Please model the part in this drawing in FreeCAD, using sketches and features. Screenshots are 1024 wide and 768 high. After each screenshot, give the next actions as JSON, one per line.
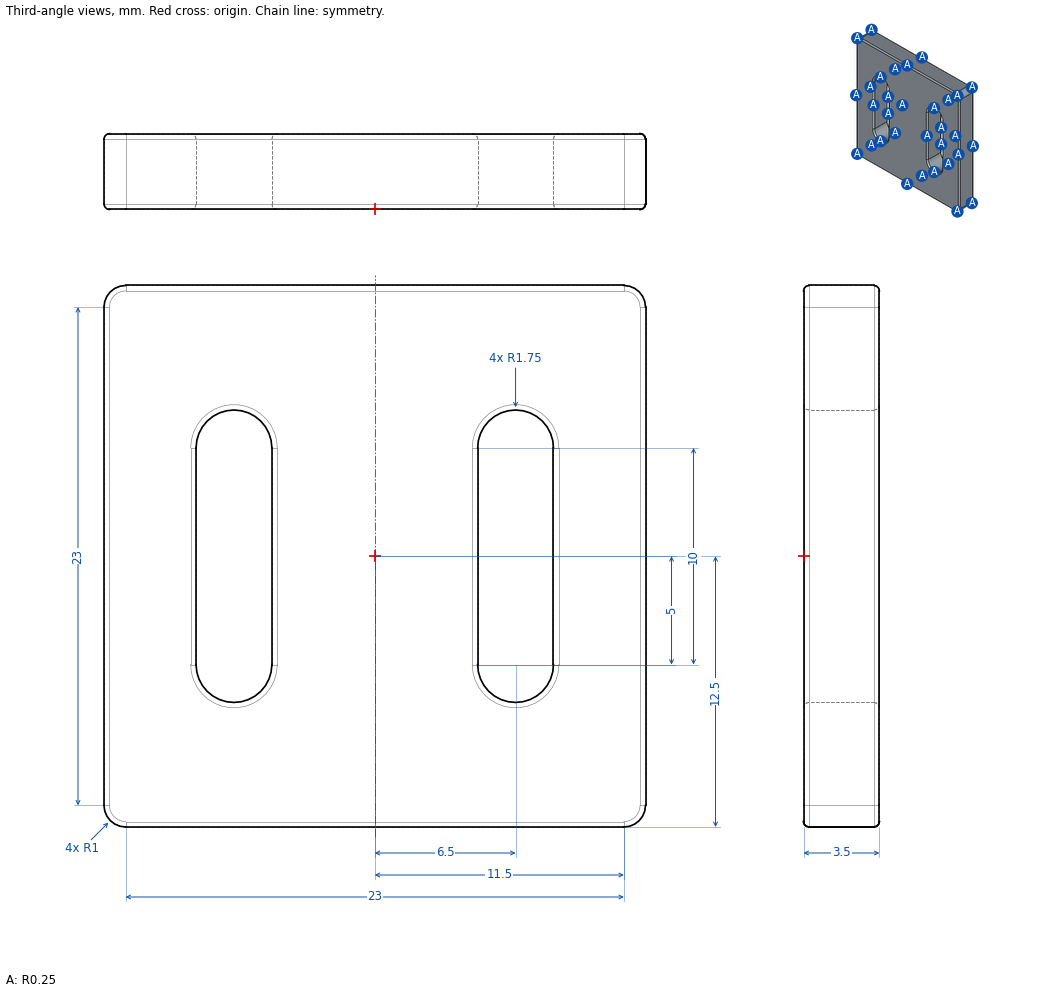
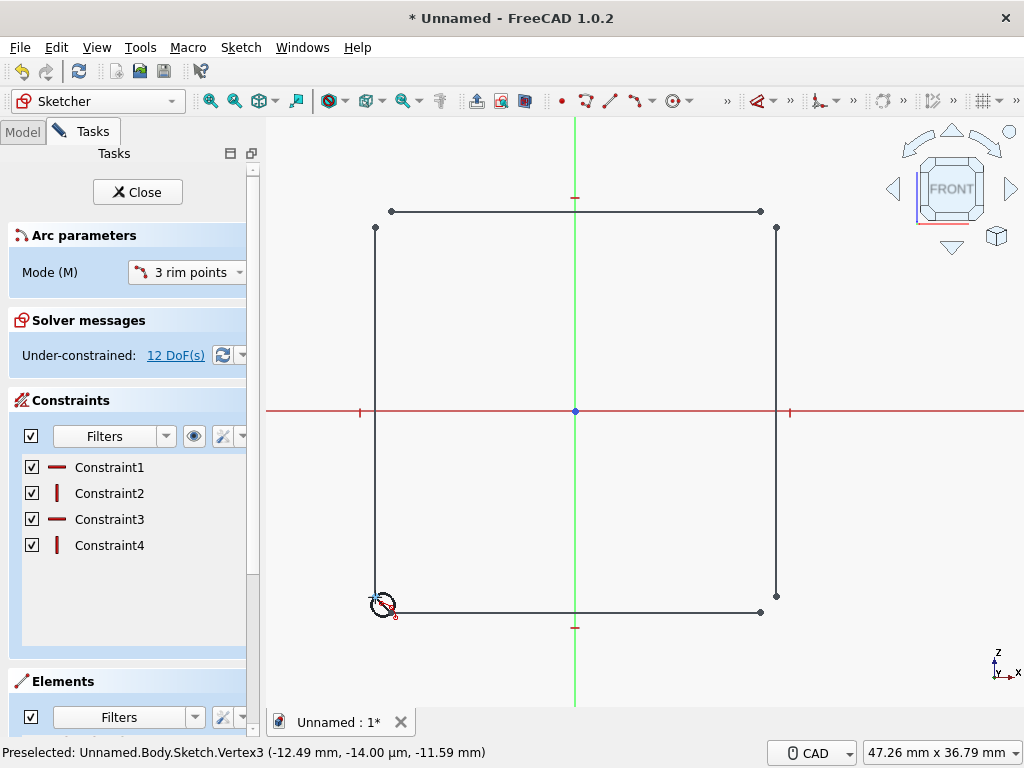
{"action": "scroll", "coordinate": [380, 607], "scroll_direction": "up", "scroll_amount": 7}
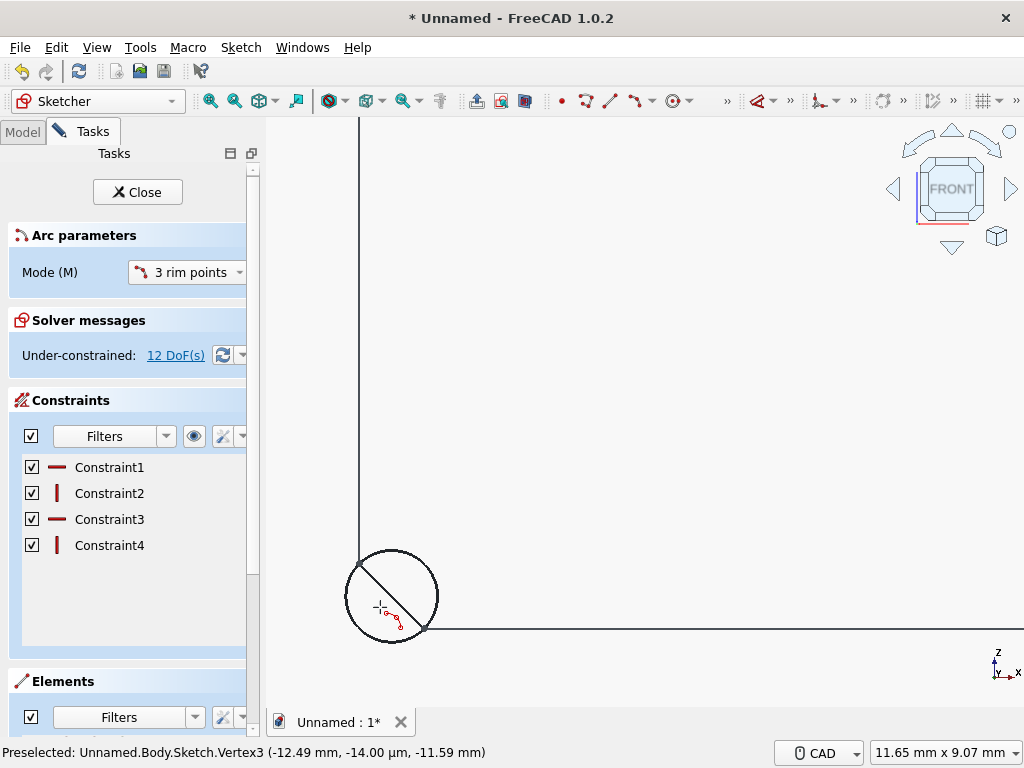
{"action": "left_click", "coordinate": [378, 604]}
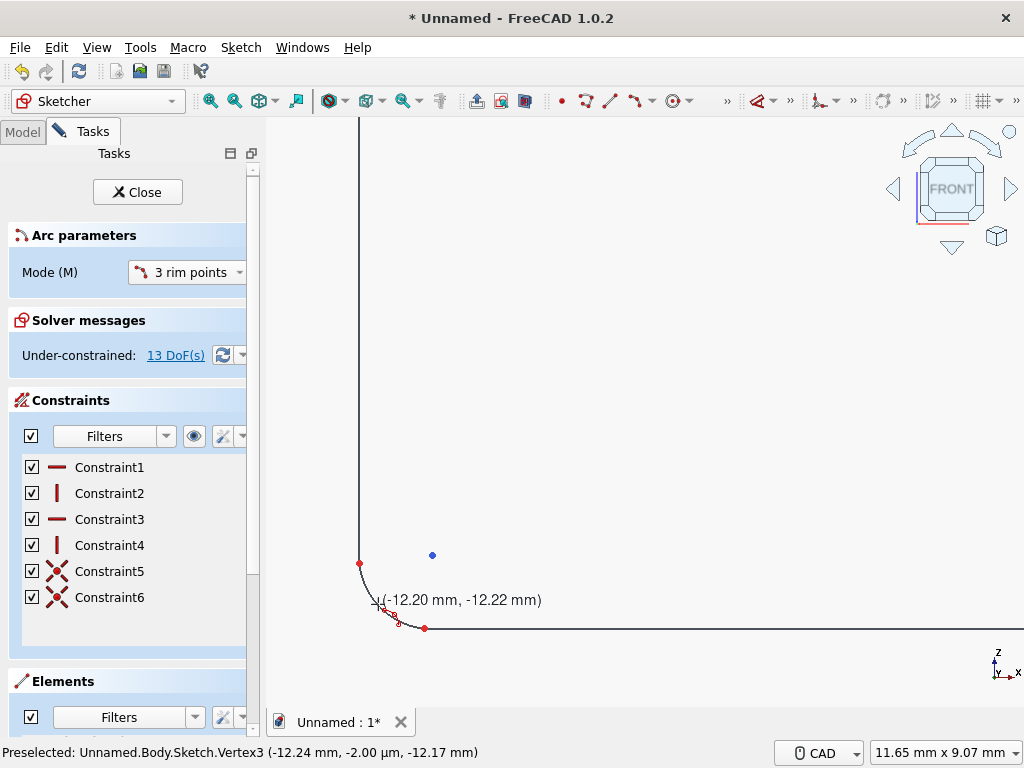
{"action": "scroll", "coordinate": [382, 609], "scroll_direction": "down", "scroll_amount": 7}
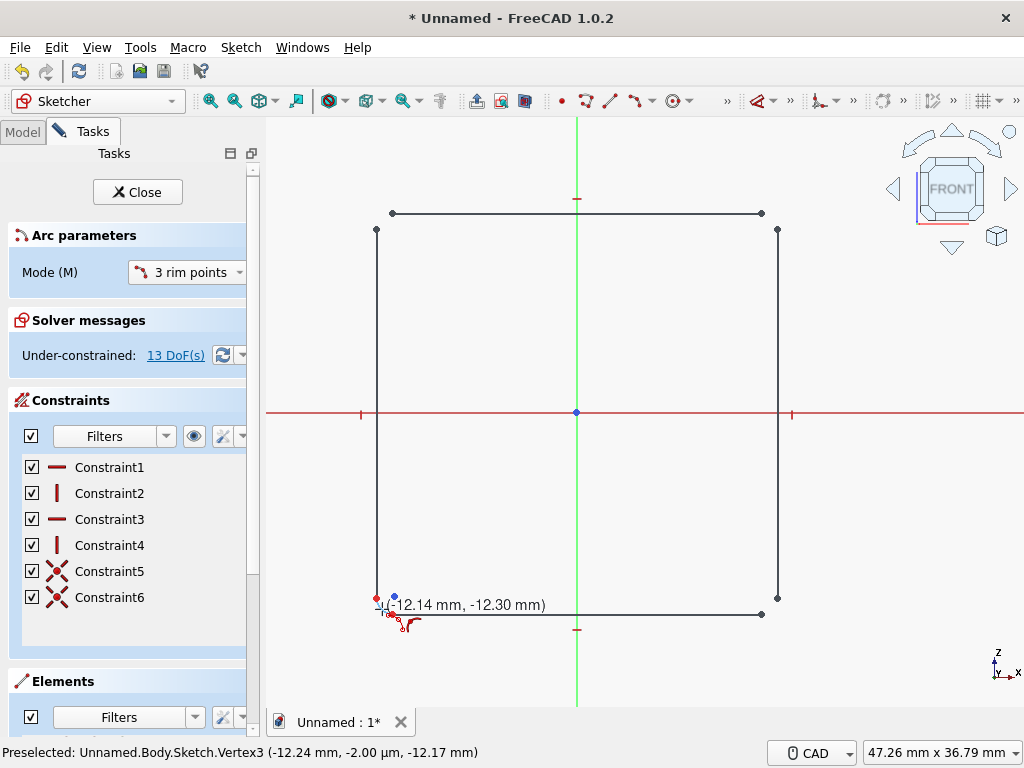
{"action": "left_click", "coordinate": [377, 230]}
{"action": "left_click", "coordinate": [393, 214]}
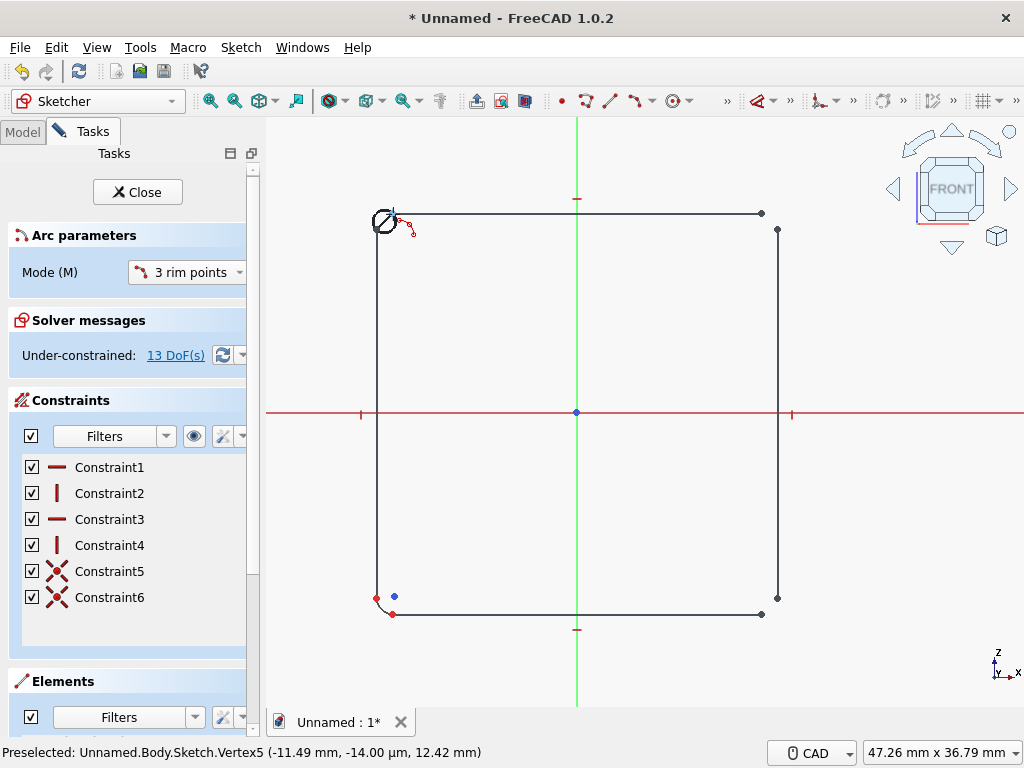
{"action": "scroll", "coordinate": [381, 217], "scroll_direction": "up", "scroll_amount": 7}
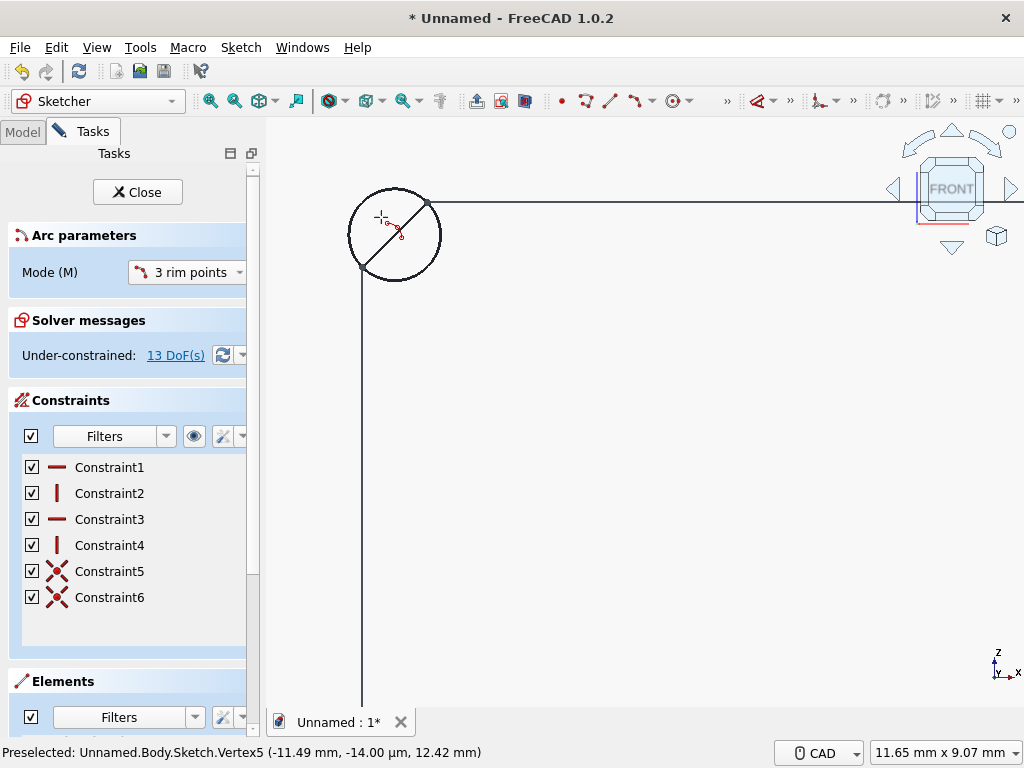
{"action": "left_click", "coordinate": [381, 216]}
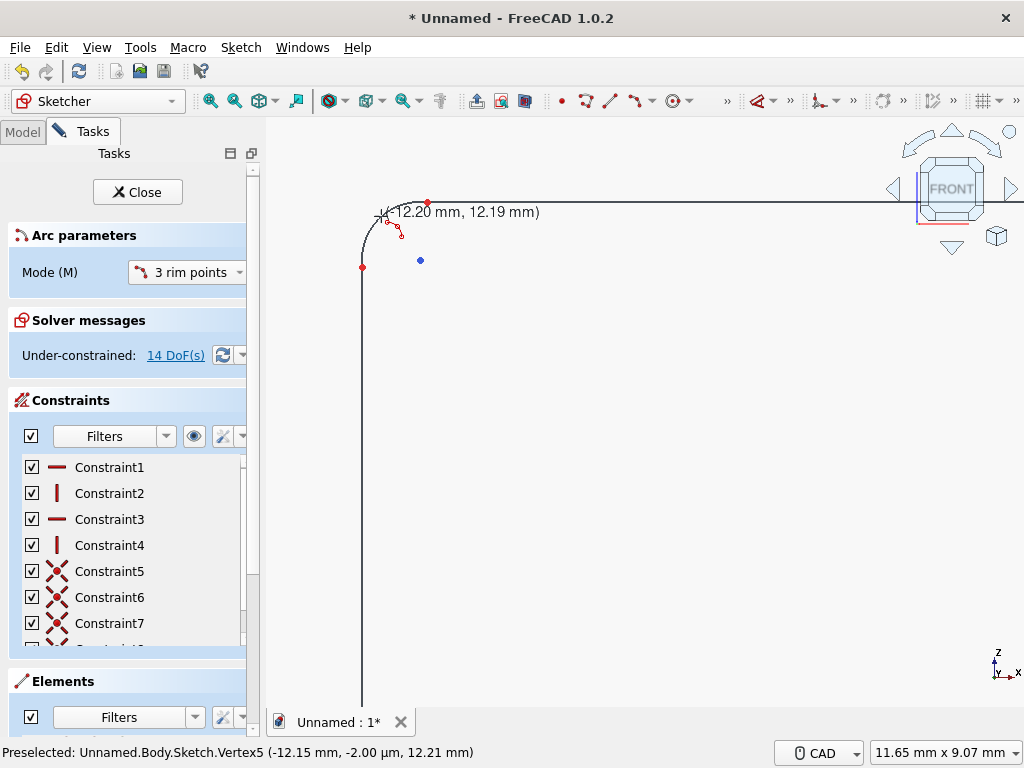
{"action": "scroll", "coordinate": [381, 216], "scroll_direction": "down", "scroll_amount": 7}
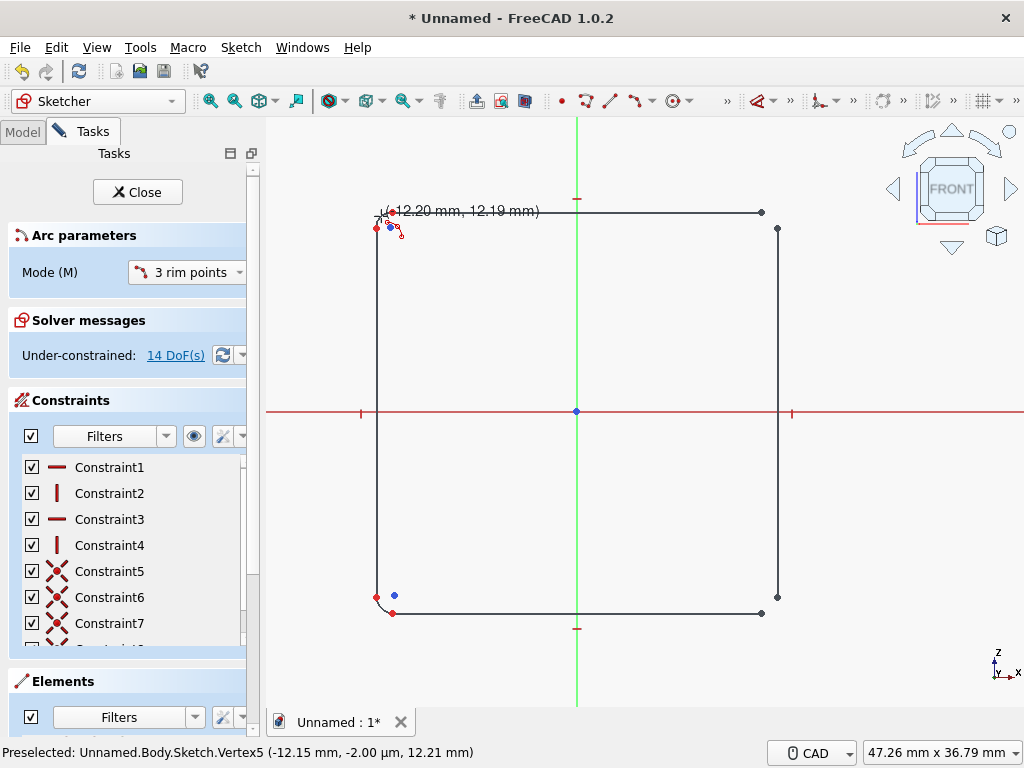
{"action": "left_click", "coordinate": [762, 213]}
{"action": "left_click", "coordinate": [778, 229]}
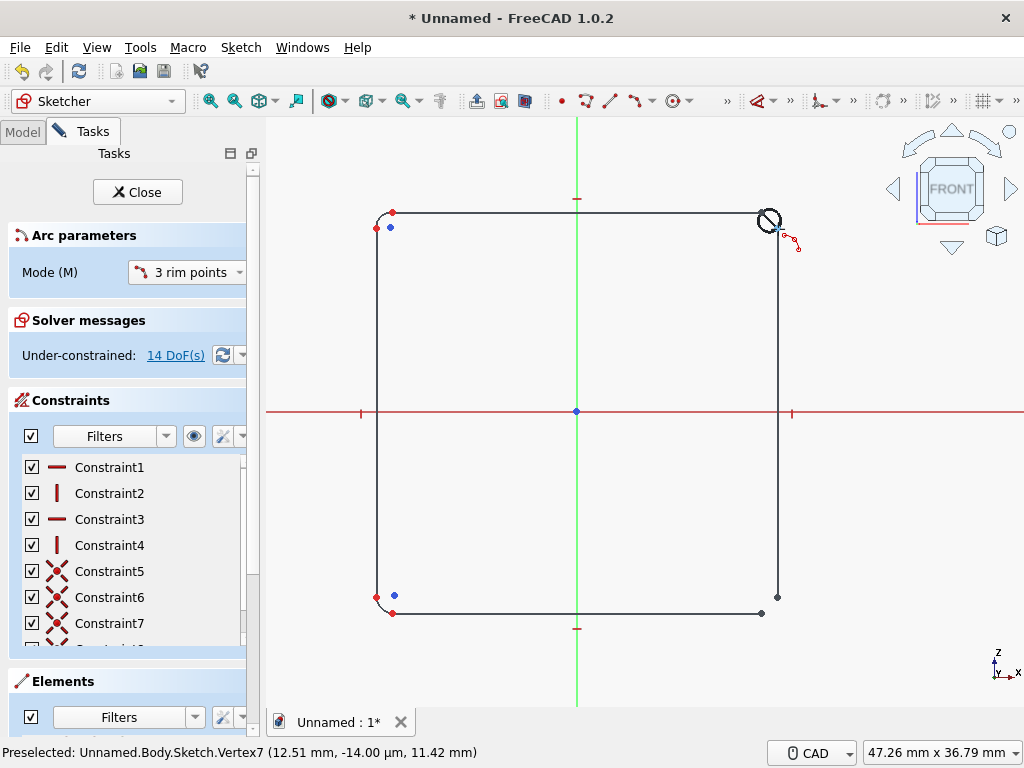
{"action": "scroll", "coordinate": [773, 216], "scroll_direction": "up", "scroll_amount": 7}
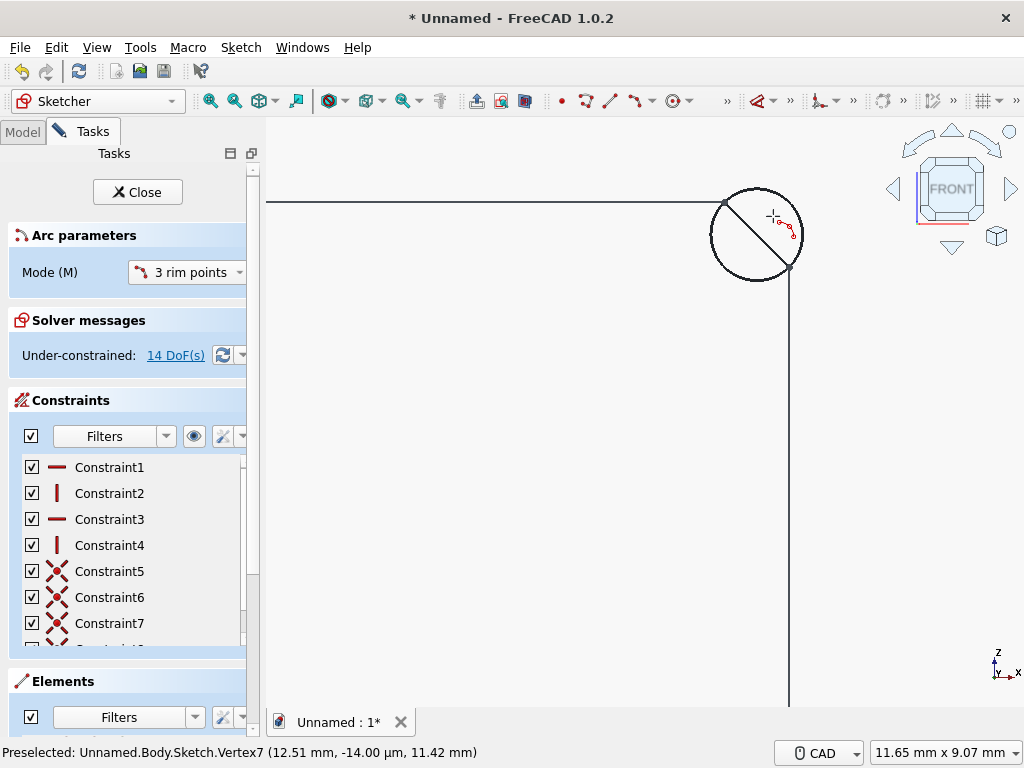
{"action": "left_click", "coordinate": [769, 216]}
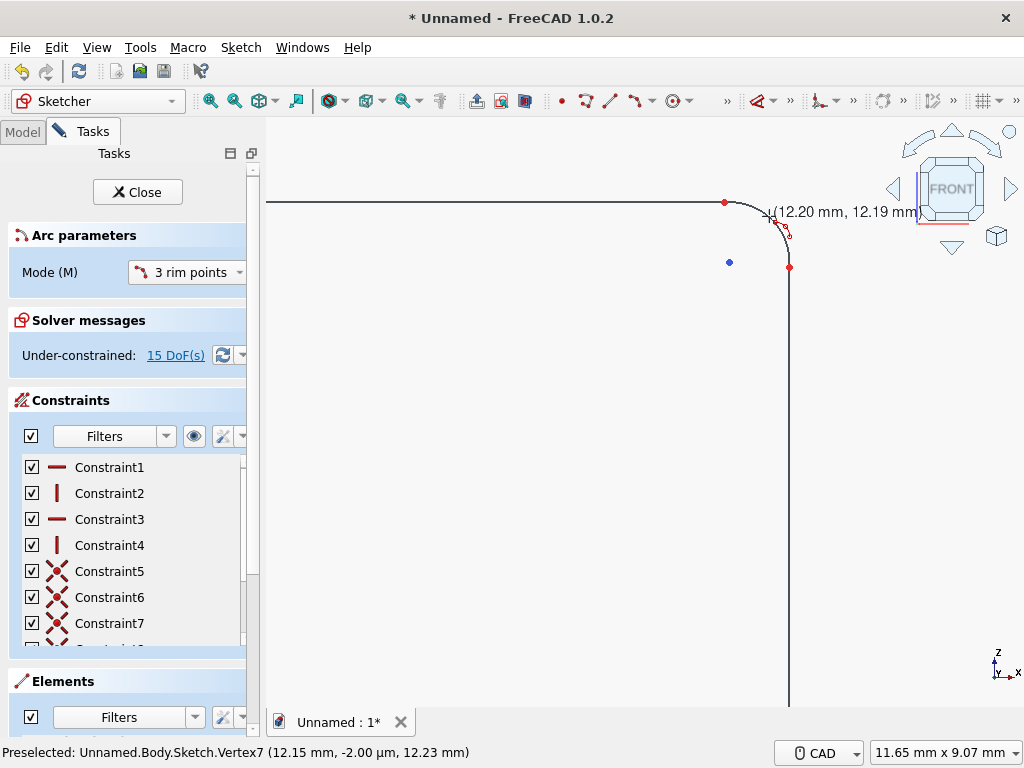
{"action": "scroll", "coordinate": [773, 216], "scroll_direction": "down", "scroll_amount": 7}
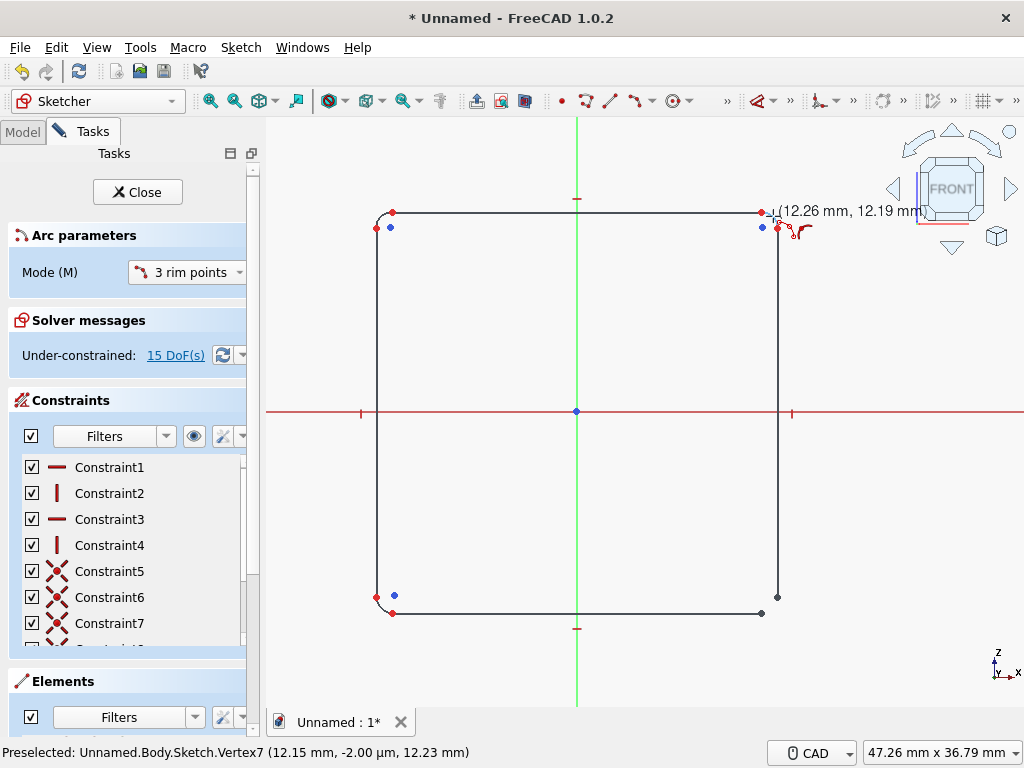
{"action": "left_click", "coordinate": [778, 598]}
{"action": "left_click", "coordinate": [762, 614]}